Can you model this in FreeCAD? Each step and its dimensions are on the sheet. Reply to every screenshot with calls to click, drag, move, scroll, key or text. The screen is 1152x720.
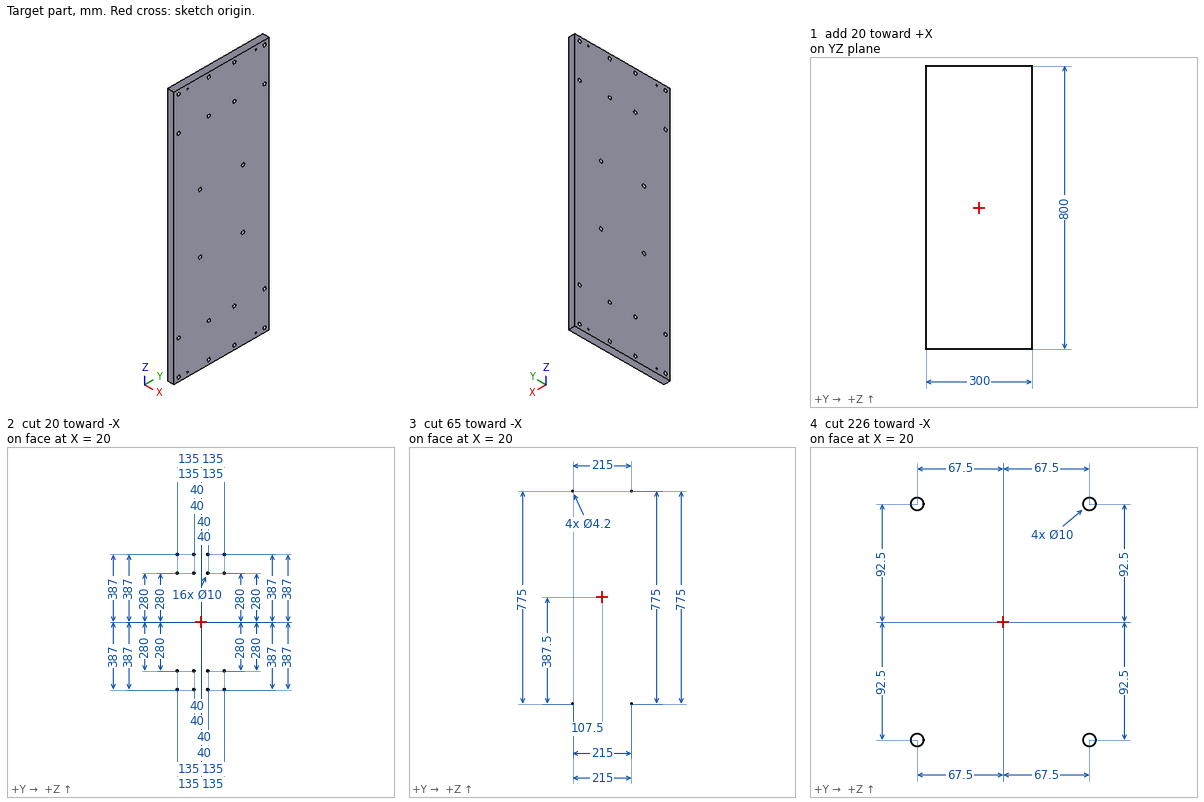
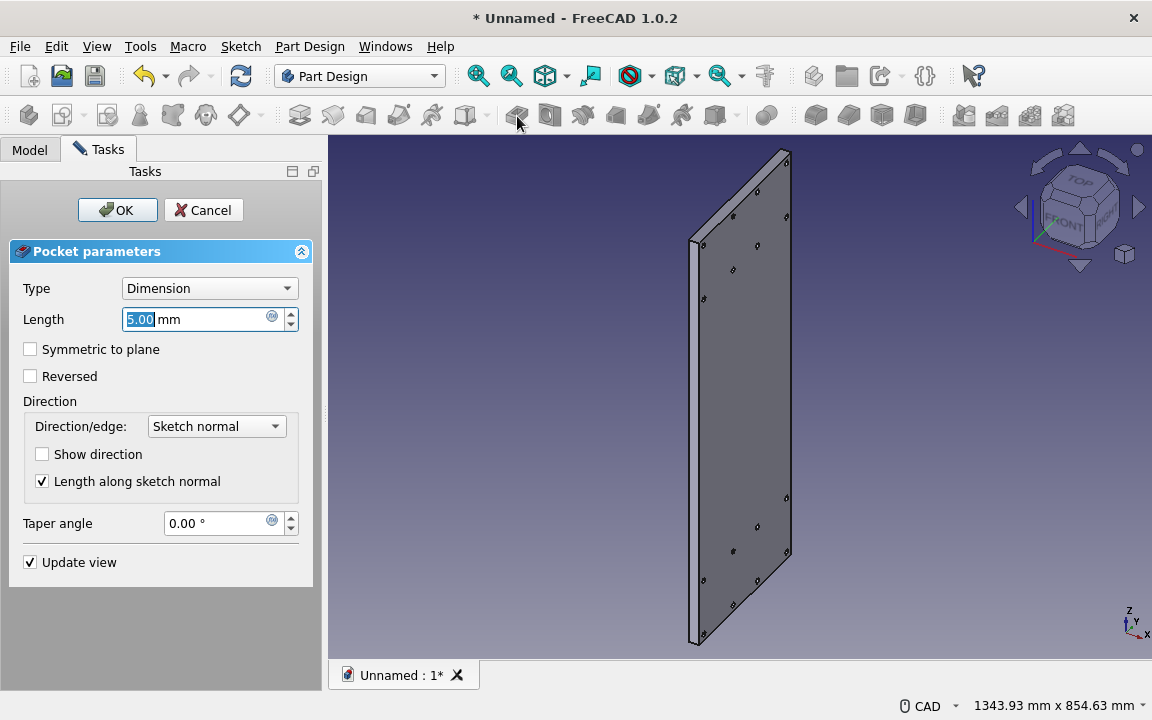
text(20)
key(Tab)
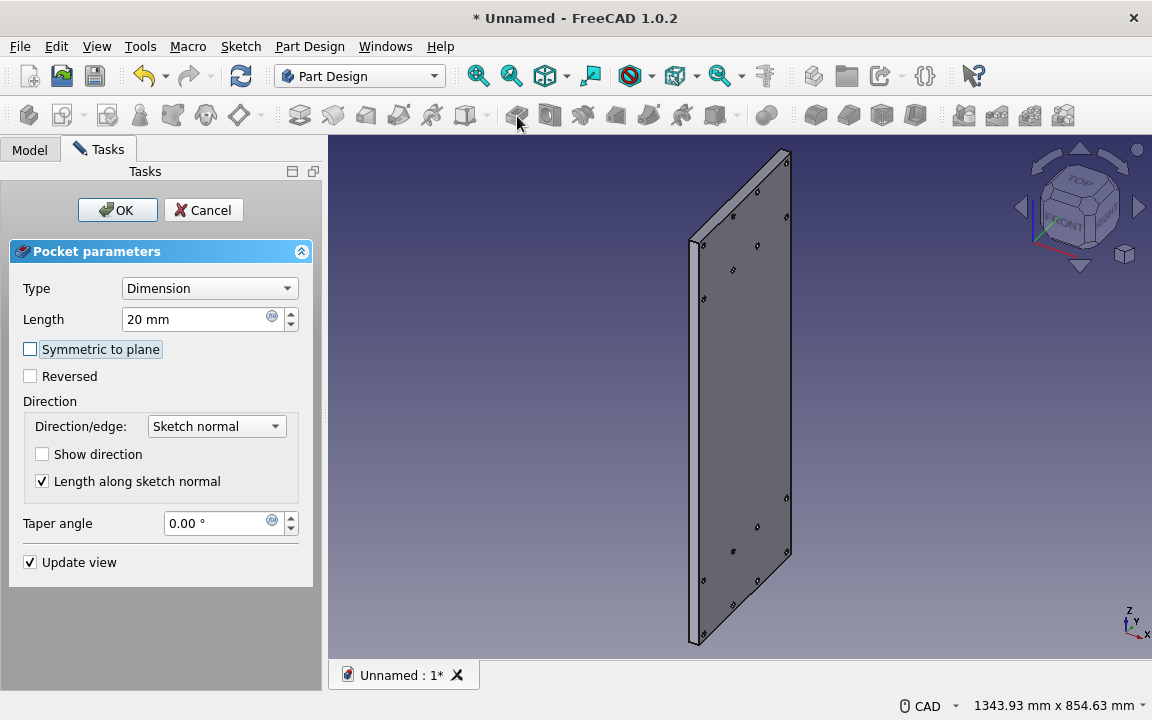
click(118, 210)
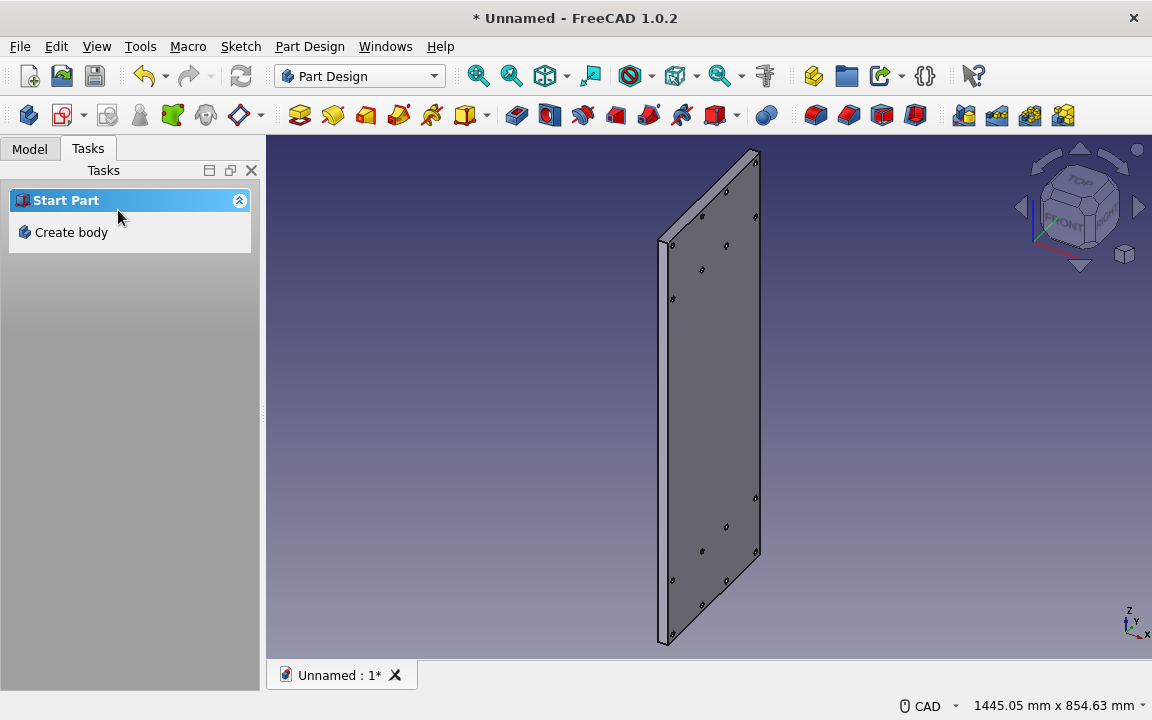
click(714, 455)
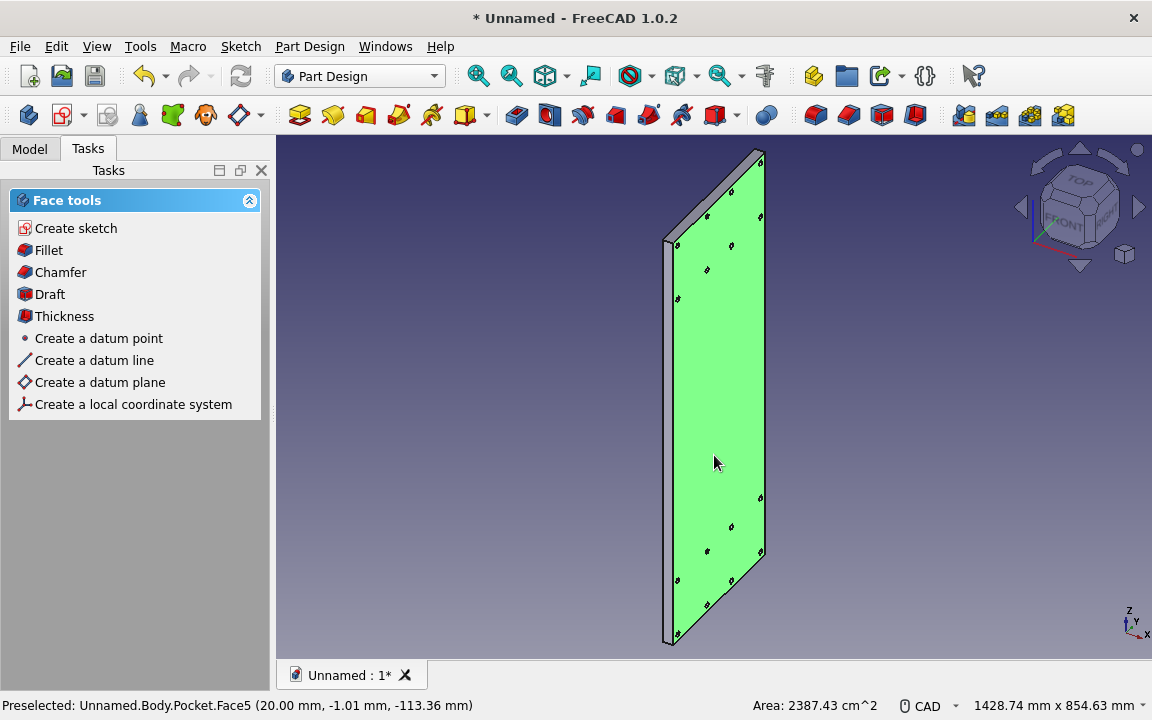
click(62, 116)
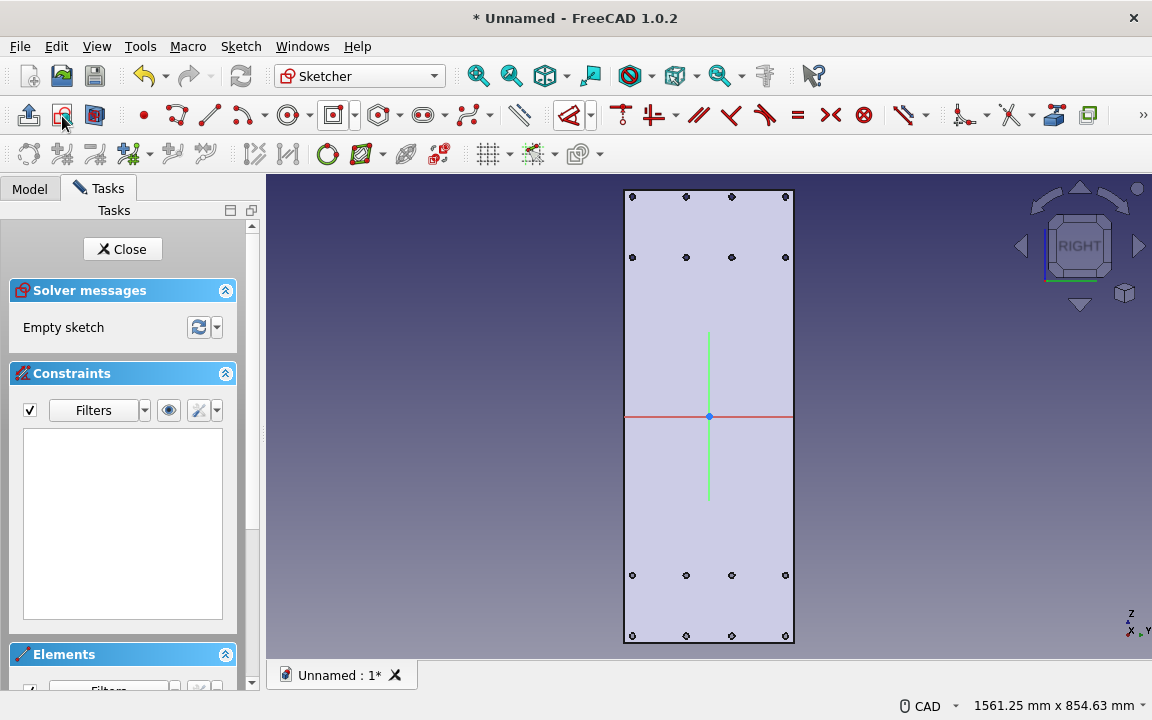
scroll(501, 416, down, 2)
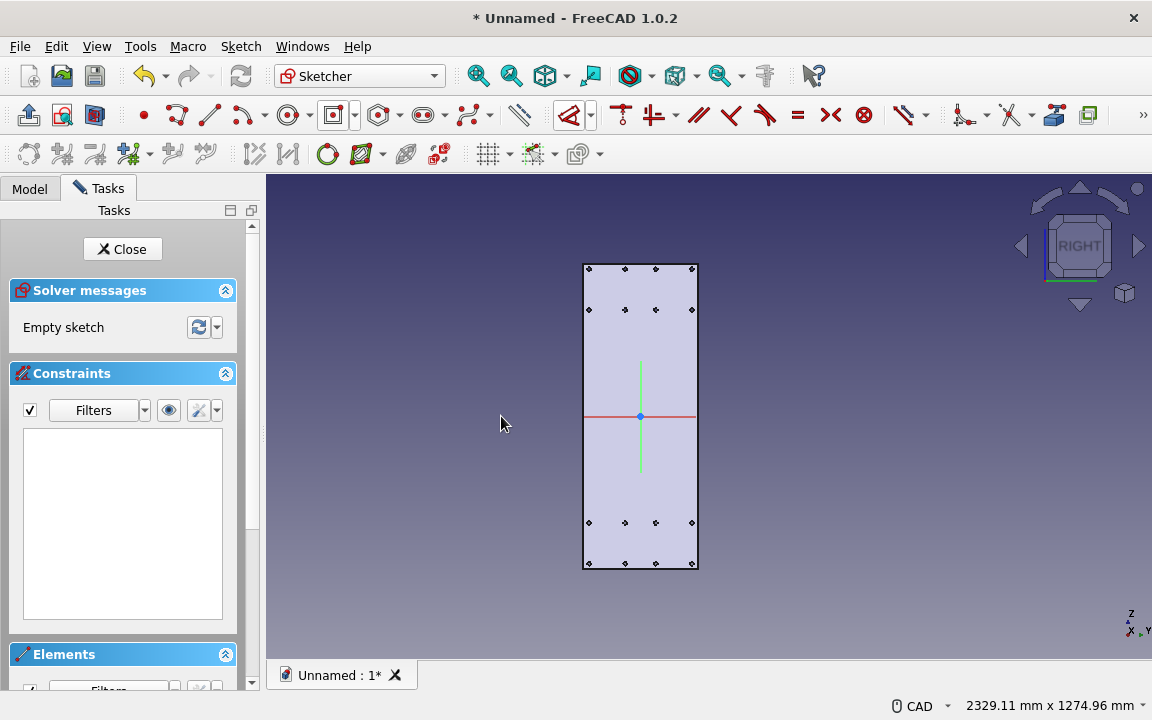
key(g)
key(c)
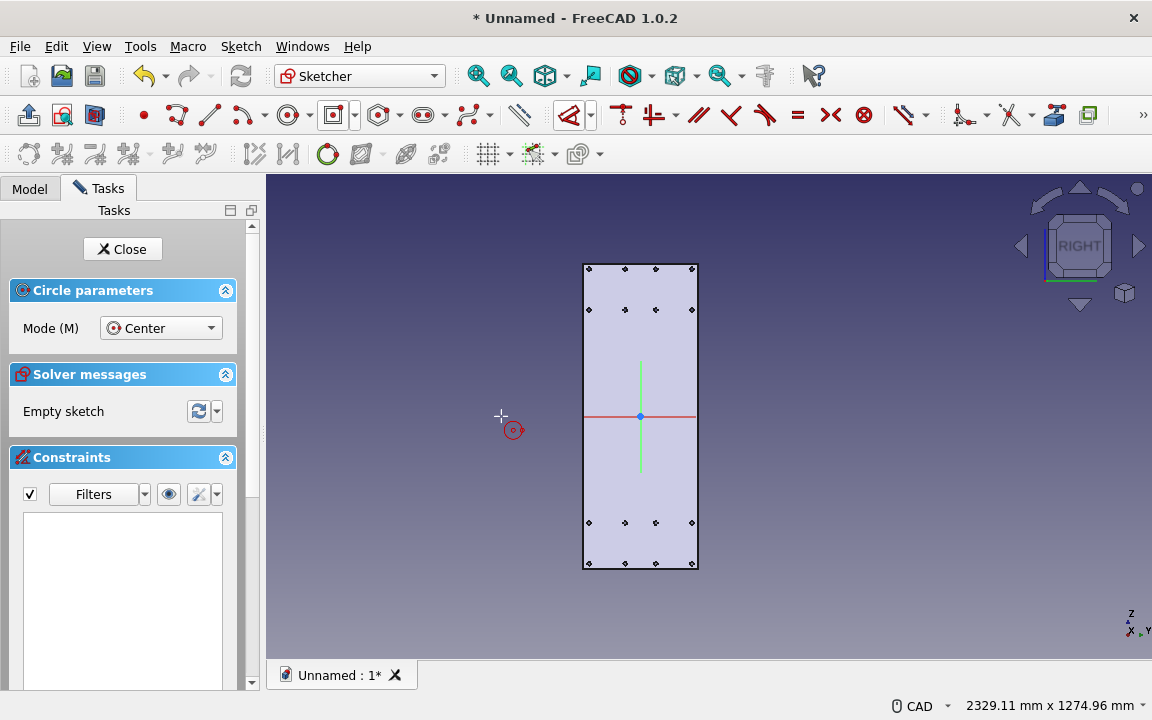
scroll(600, 564, up, 17)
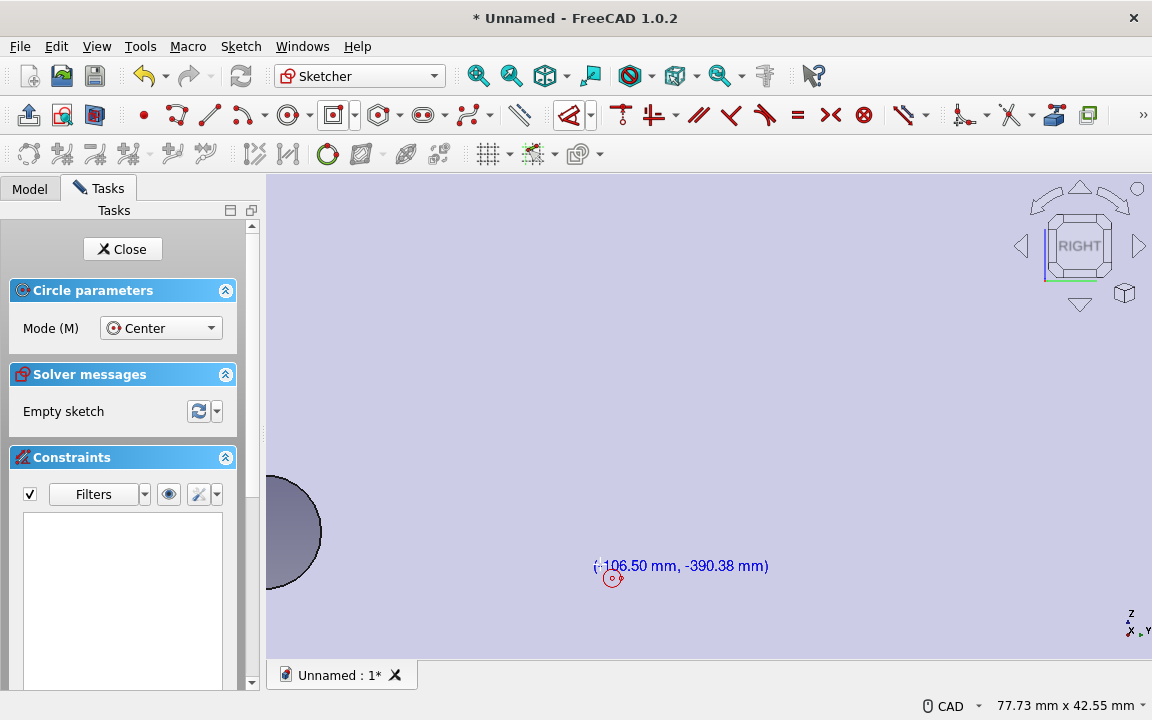
scroll(591, 599, down, 16)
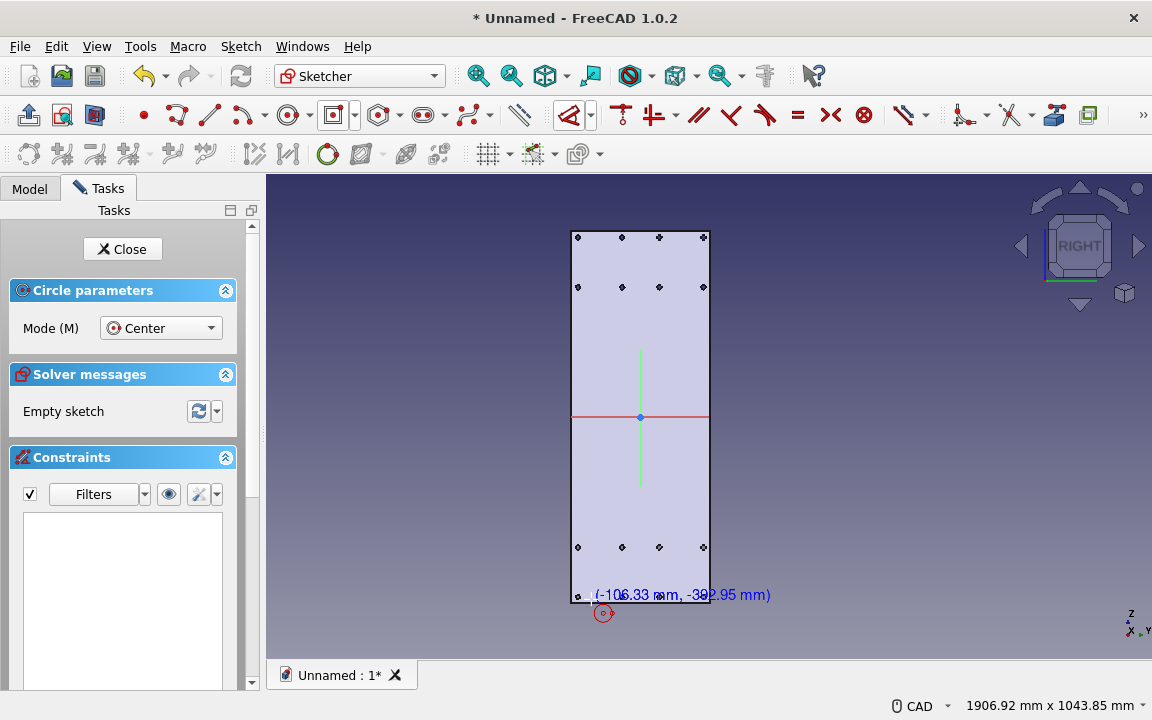
click(591, 597)
move(592, 597)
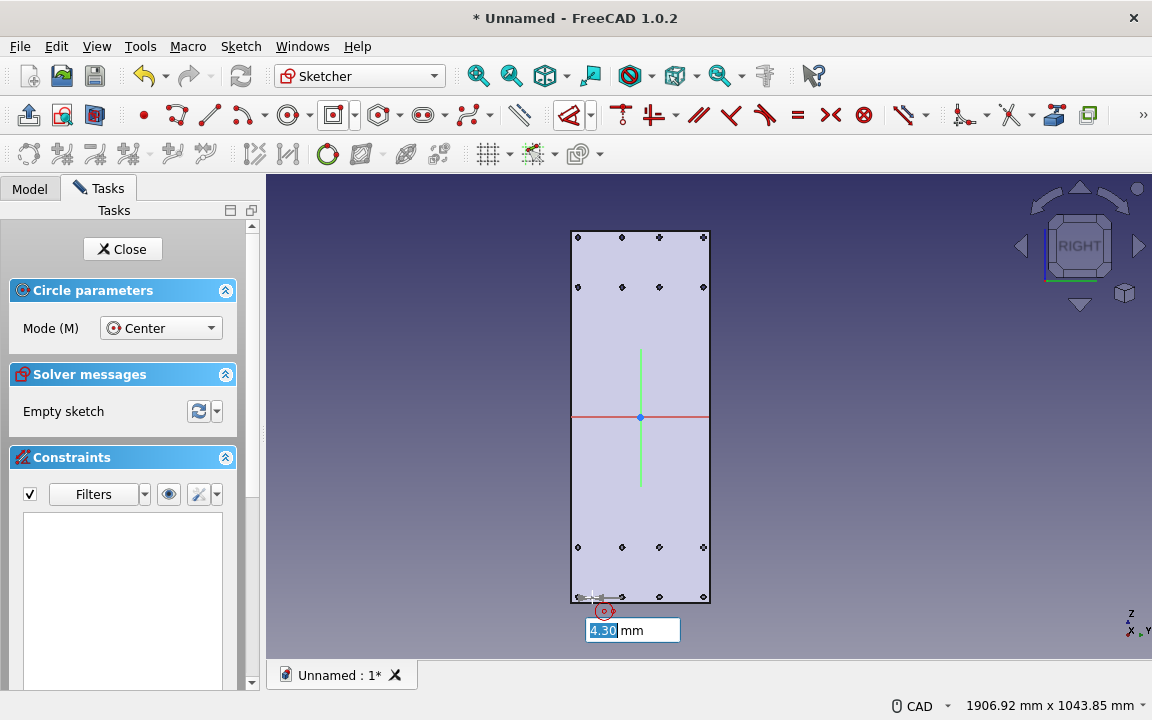
text(4.2)
key(Return)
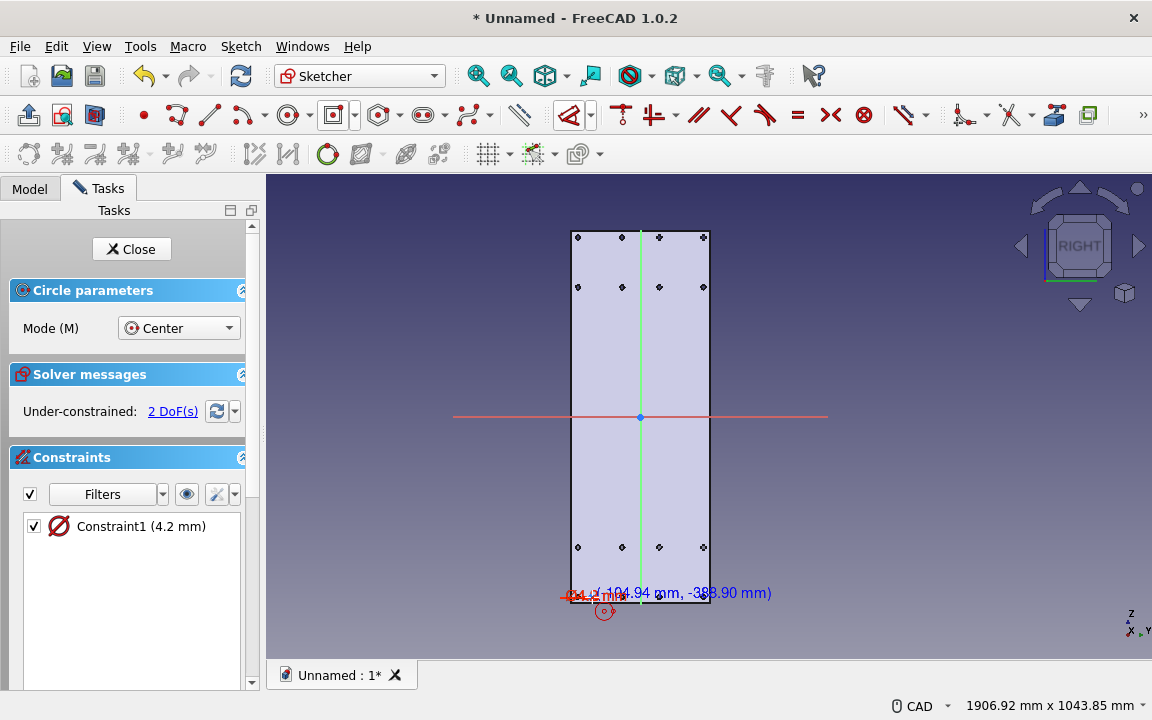
scroll(691, 597, up, 16)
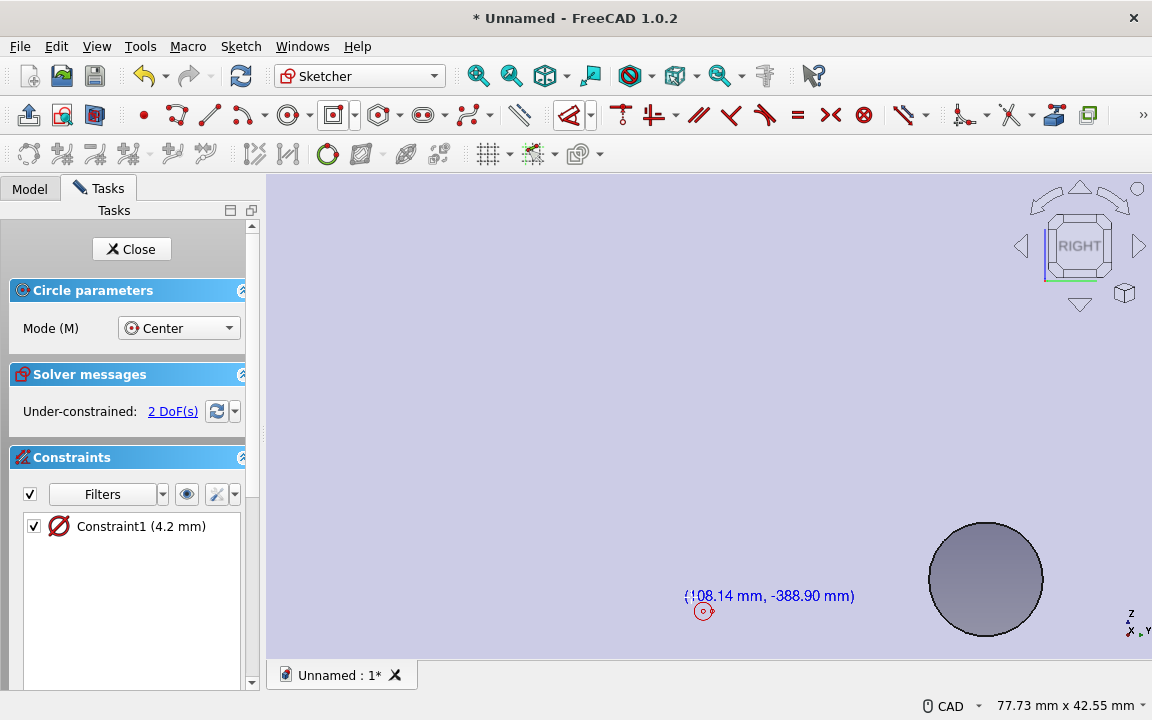
scroll(691, 597, down, 16)